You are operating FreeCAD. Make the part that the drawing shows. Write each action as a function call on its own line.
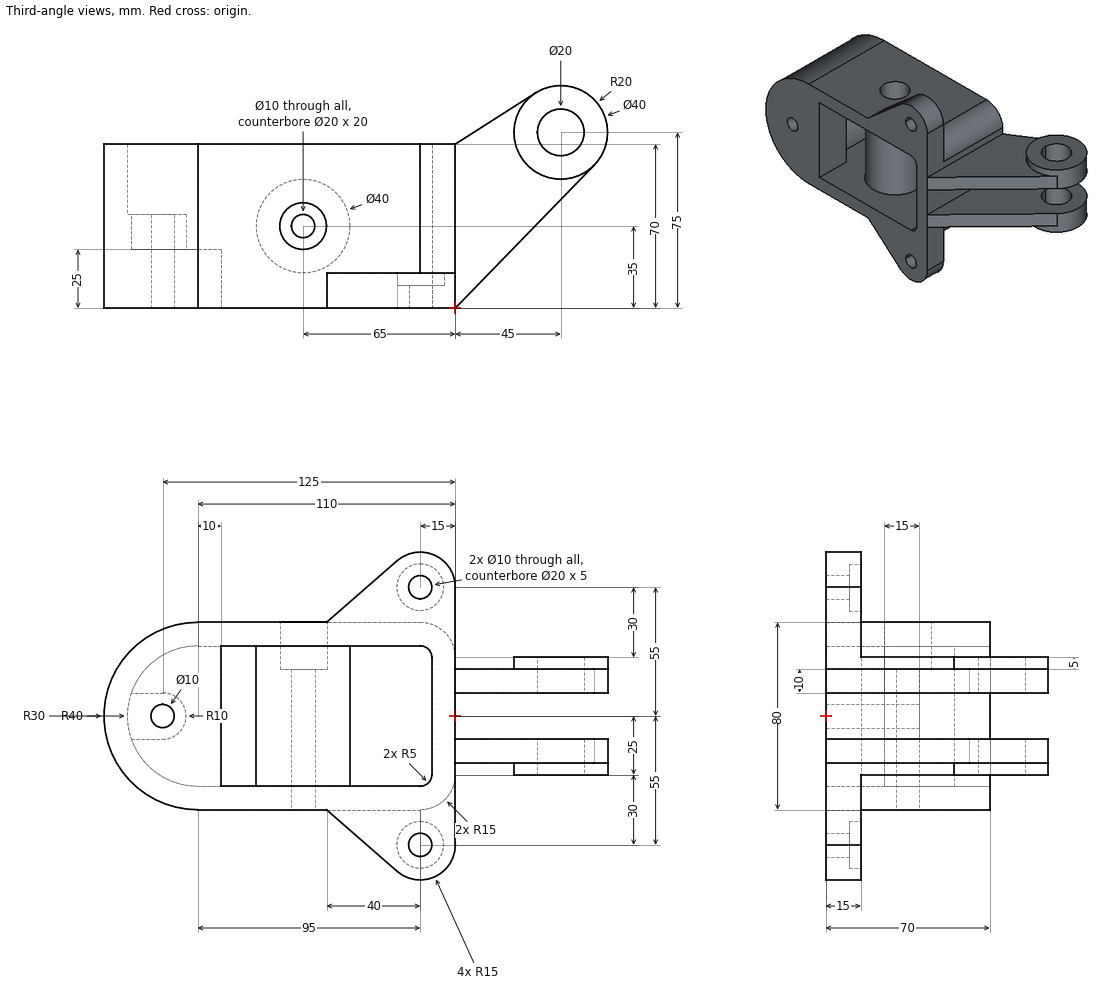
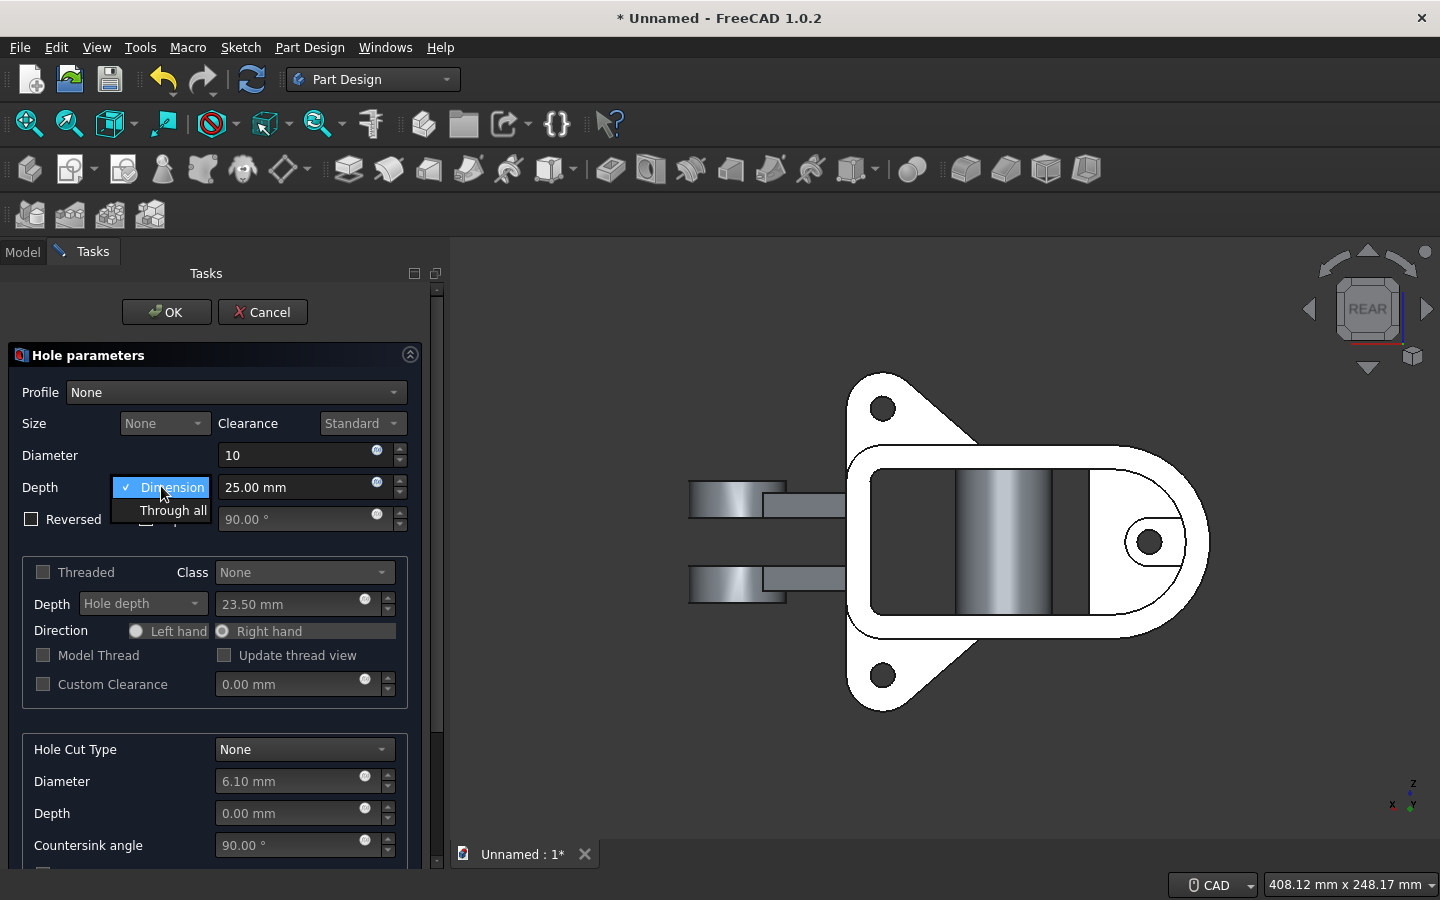
click(160, 510)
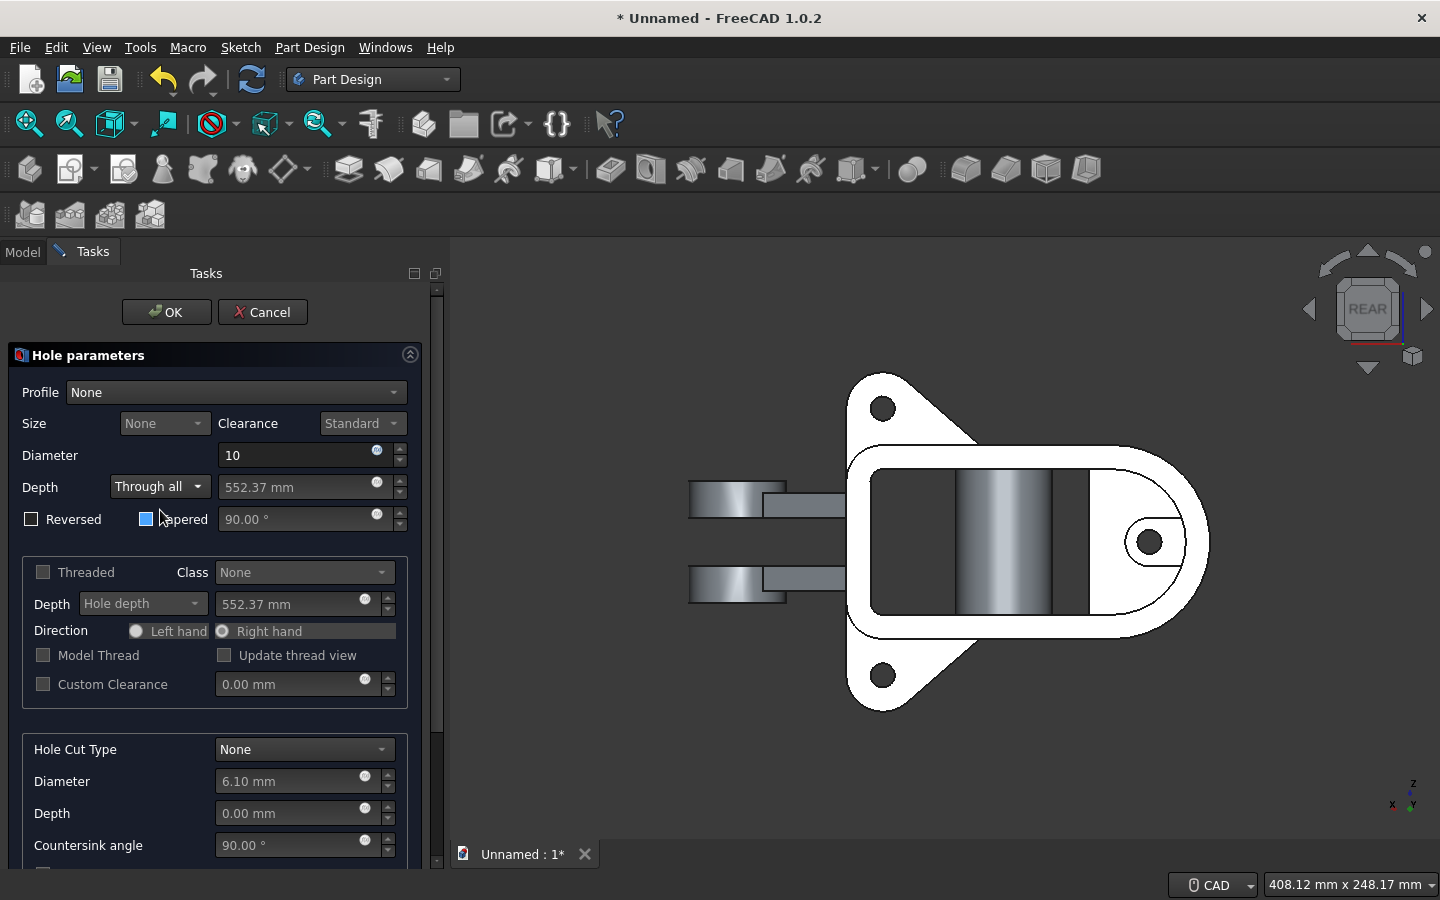
click(306, 750)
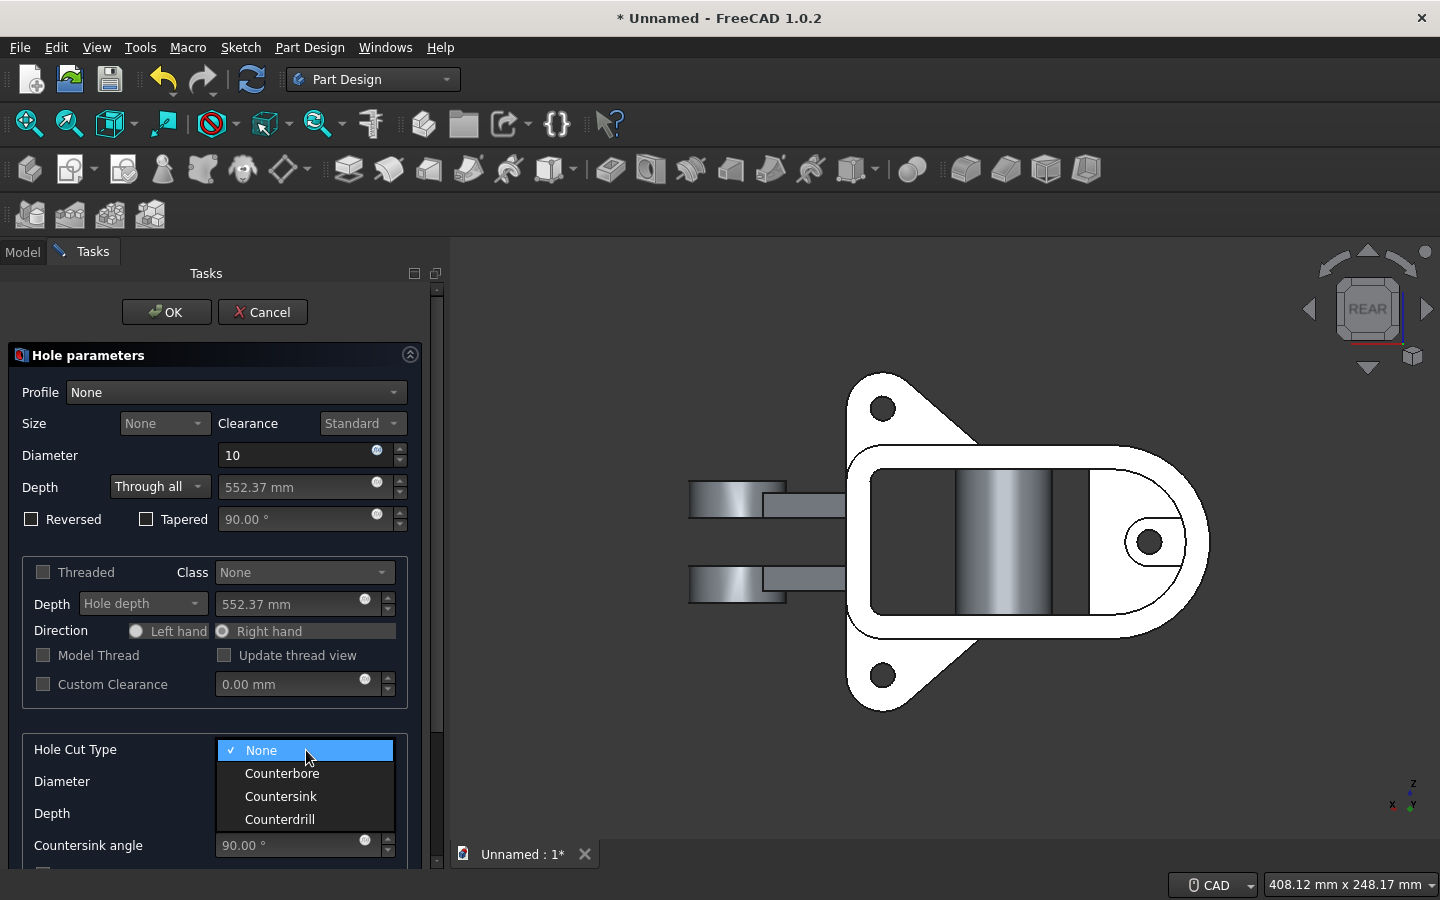
click(304, 774)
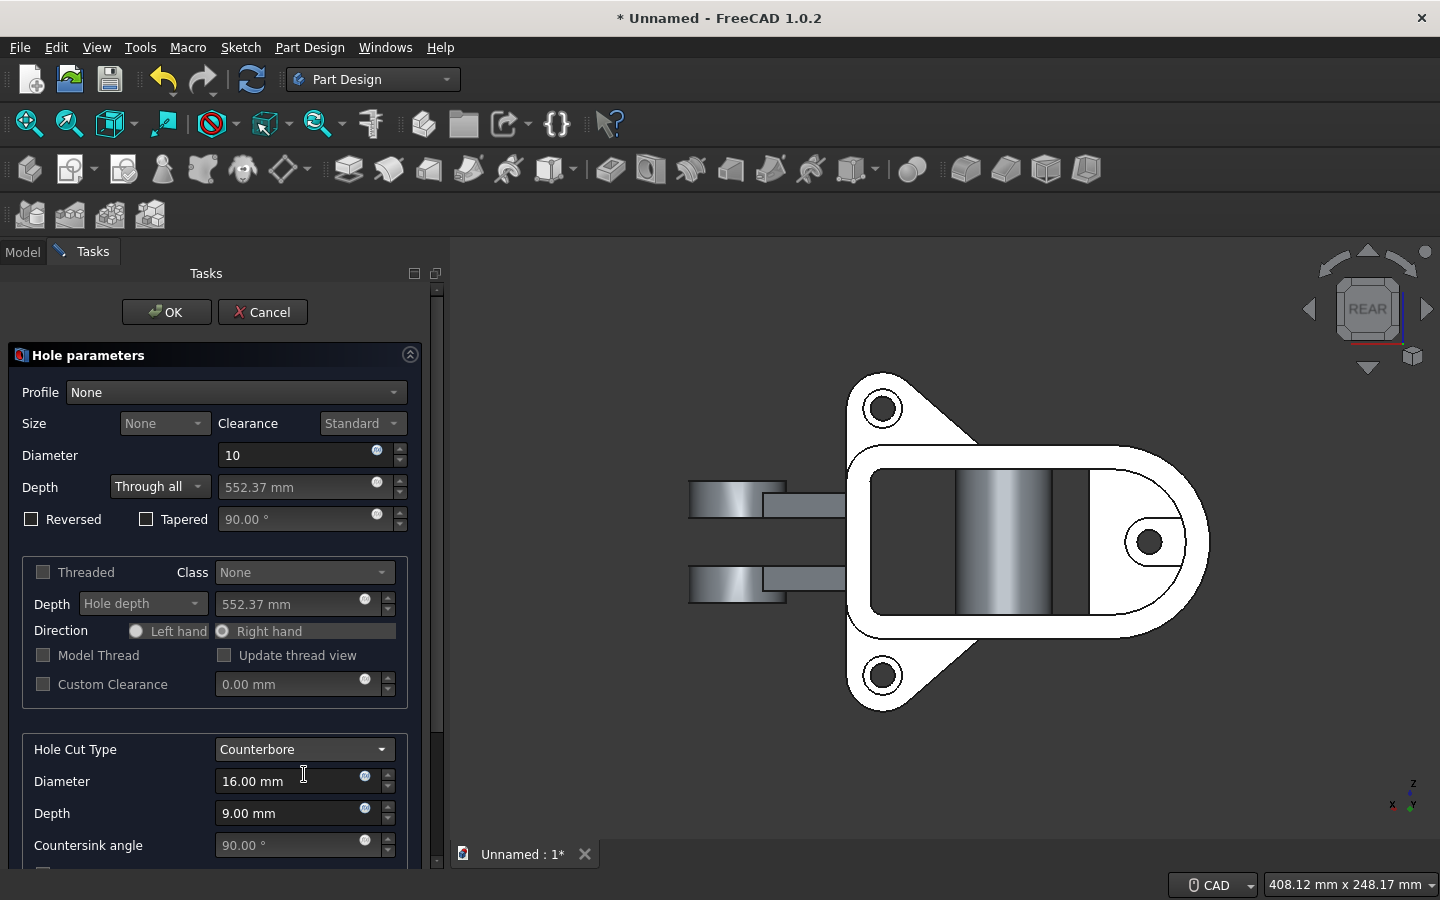
triple_click(298, 781)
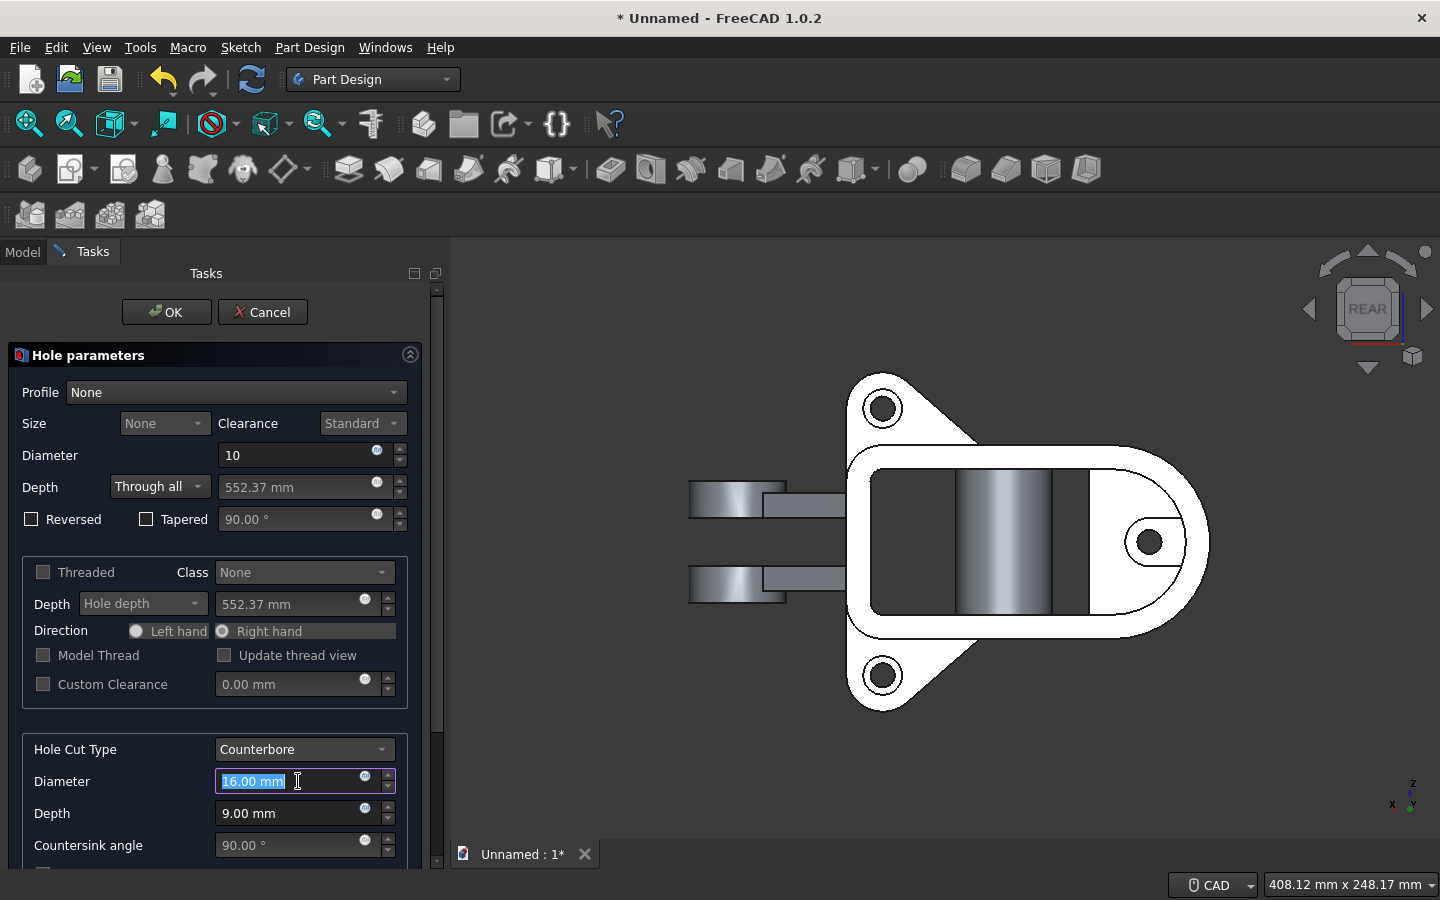
text(20)
key(Tab)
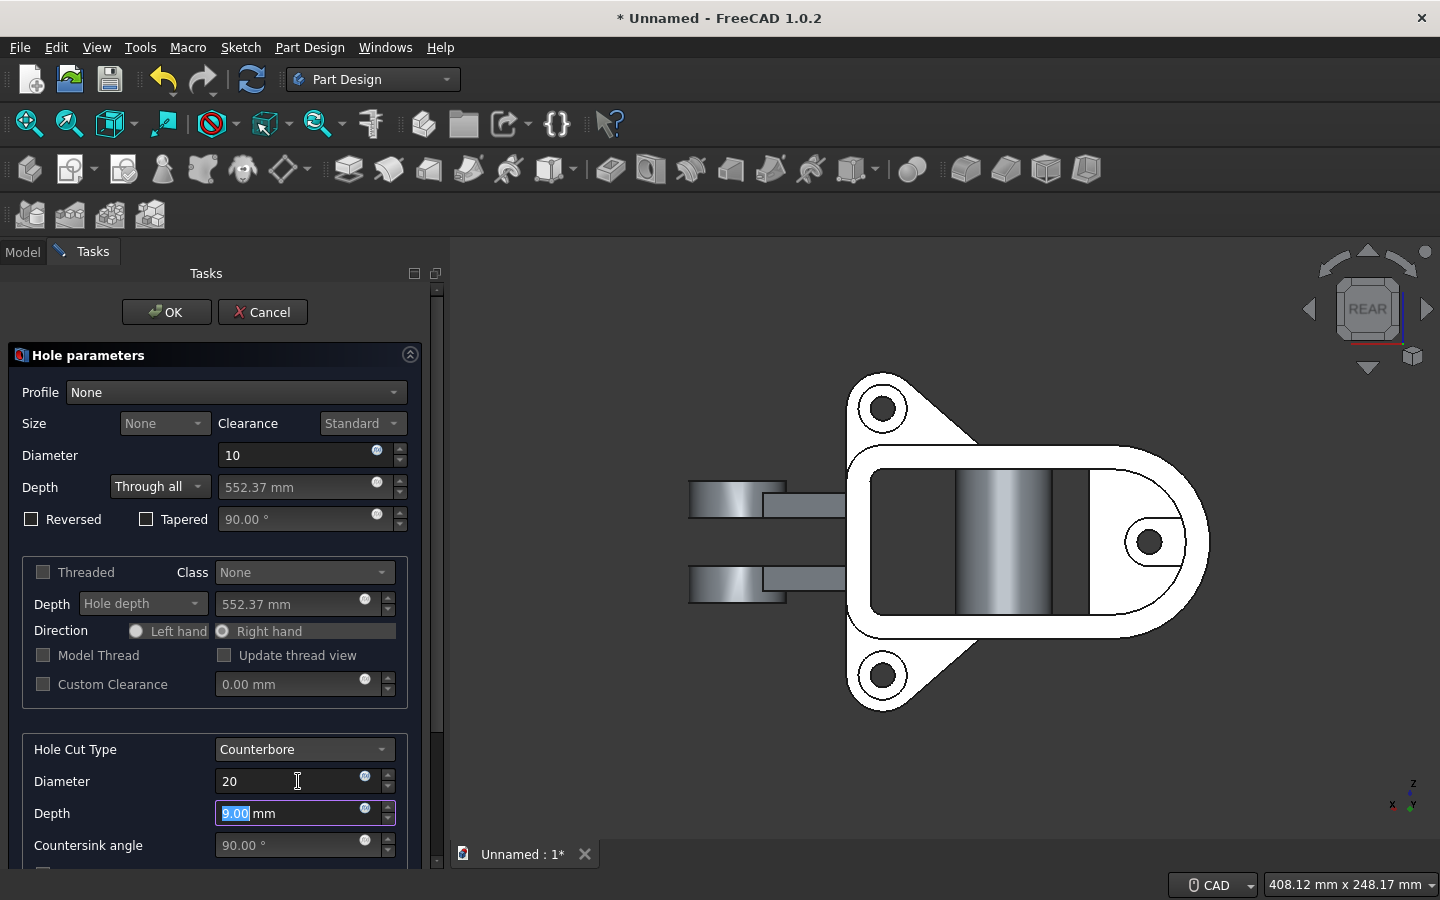
text(5)
key(Tab)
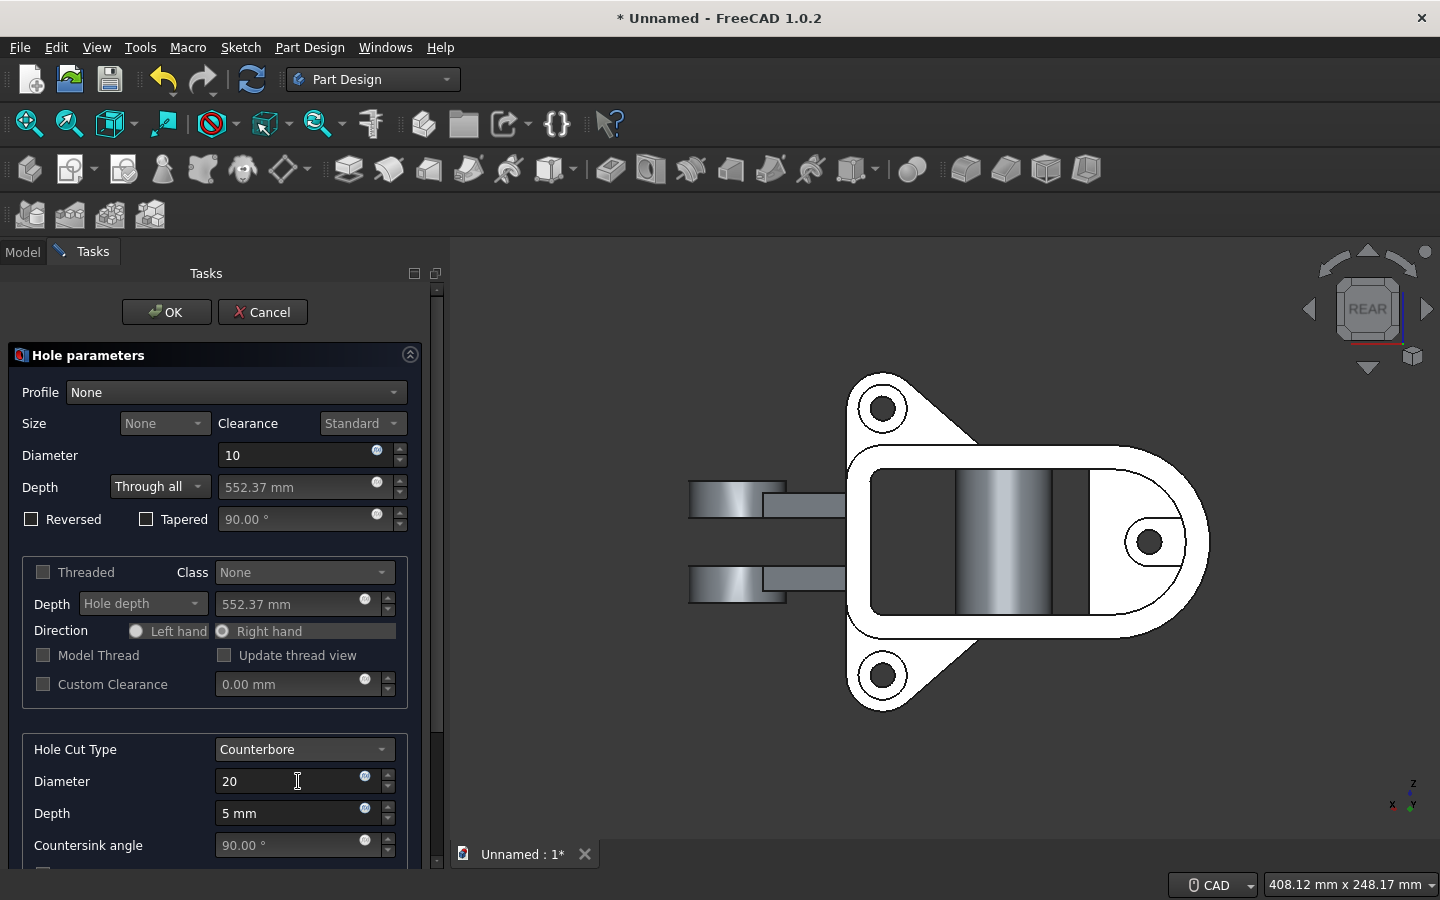
click(167, 312)